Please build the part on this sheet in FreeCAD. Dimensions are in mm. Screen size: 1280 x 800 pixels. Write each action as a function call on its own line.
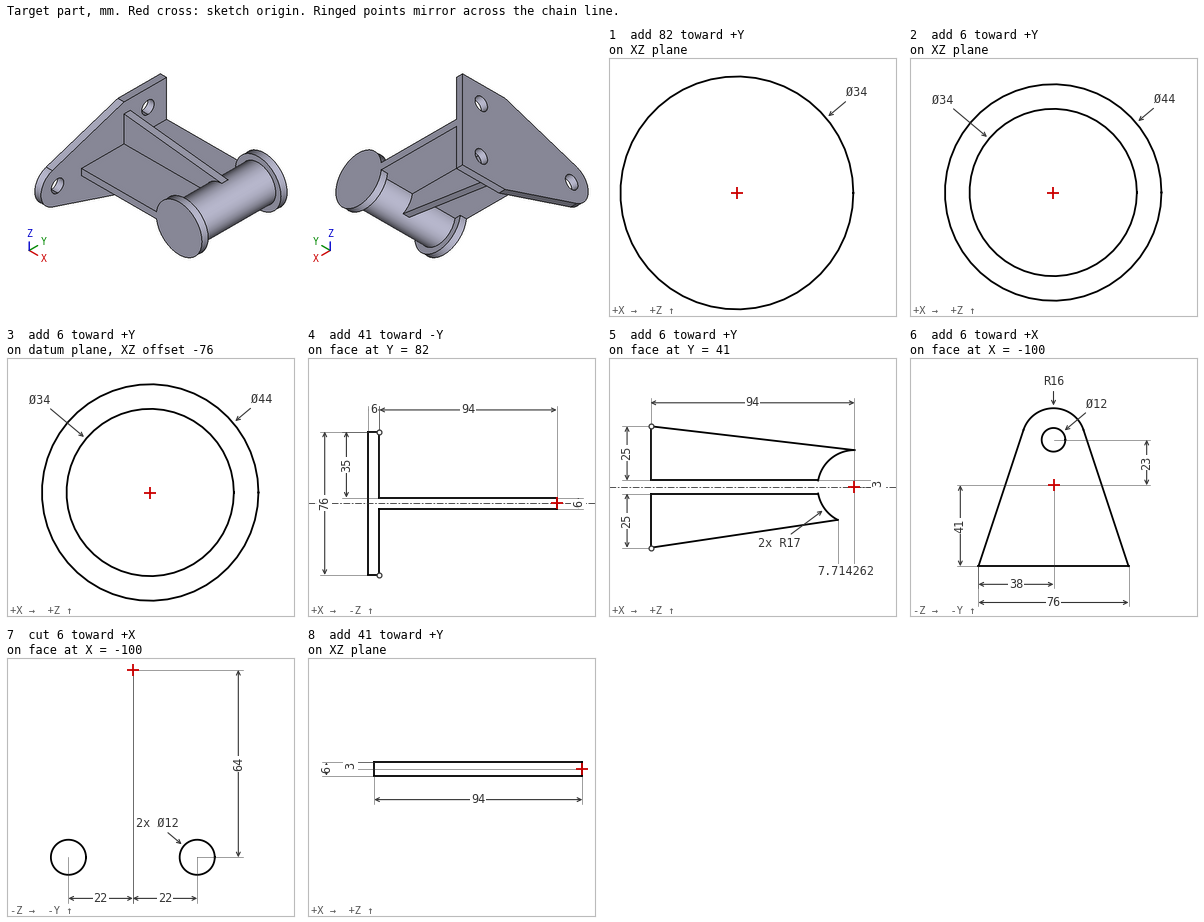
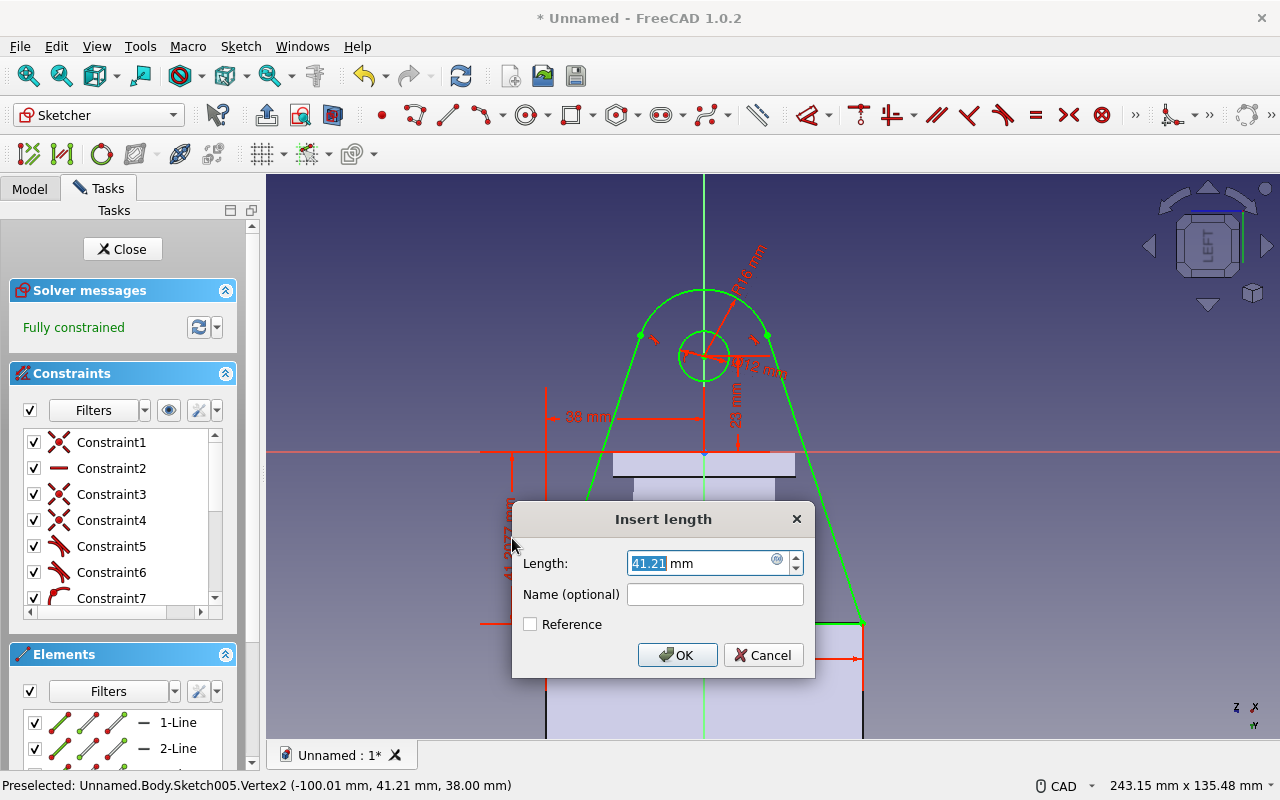
text(41)
key(Return)
key(Escape)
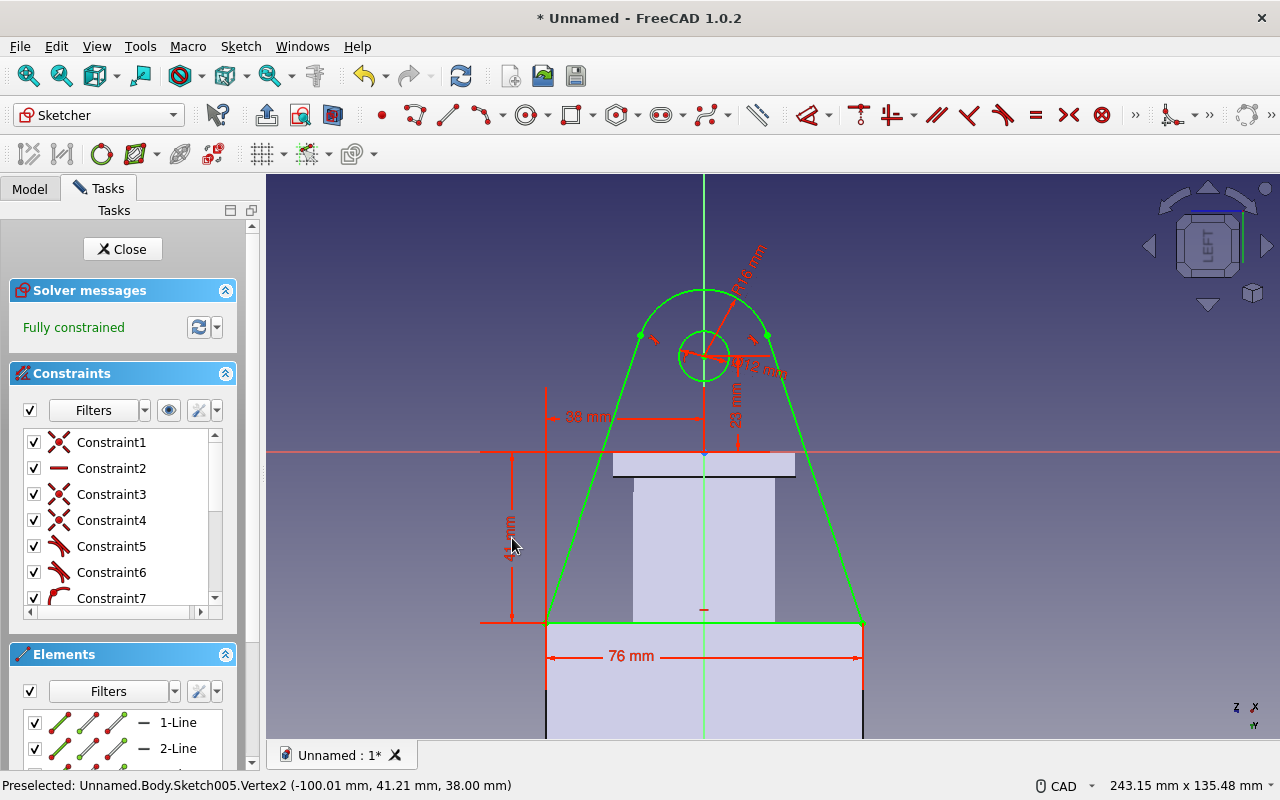
click(123, 249)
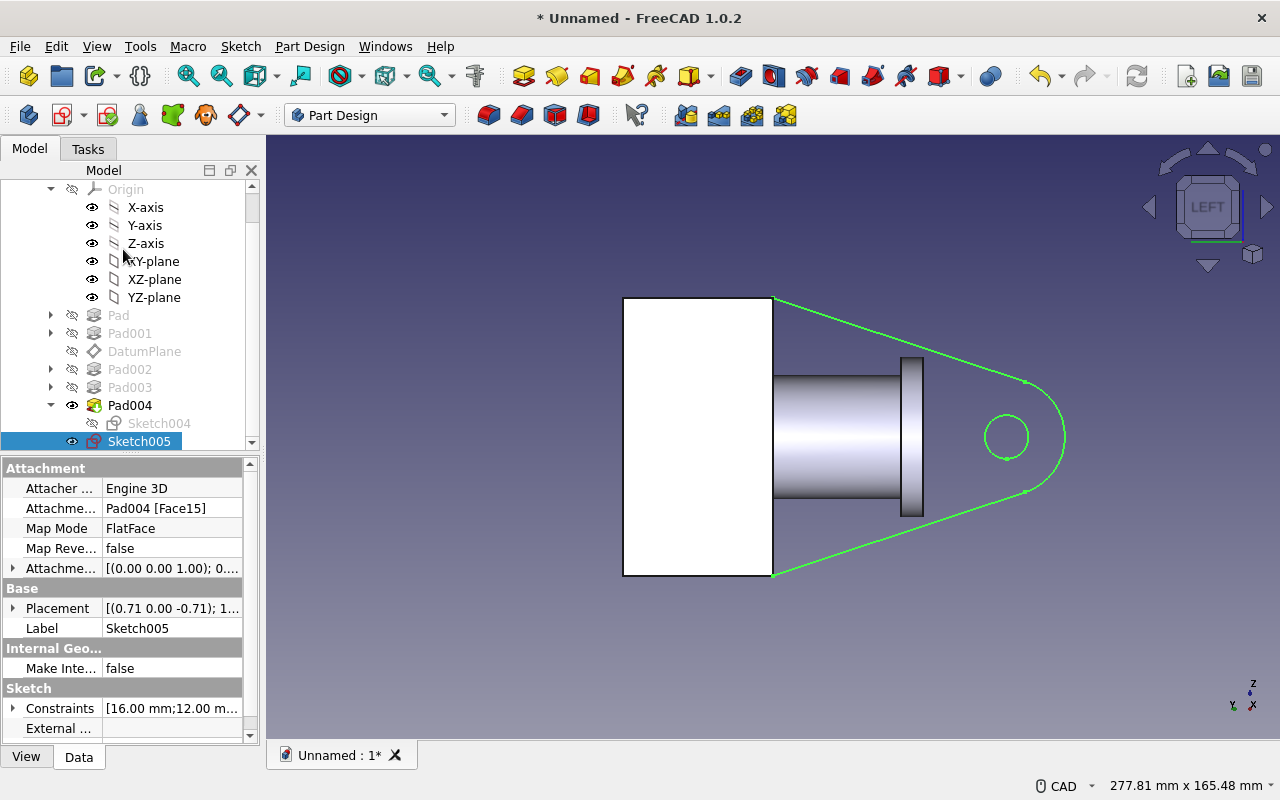
click(524, 76)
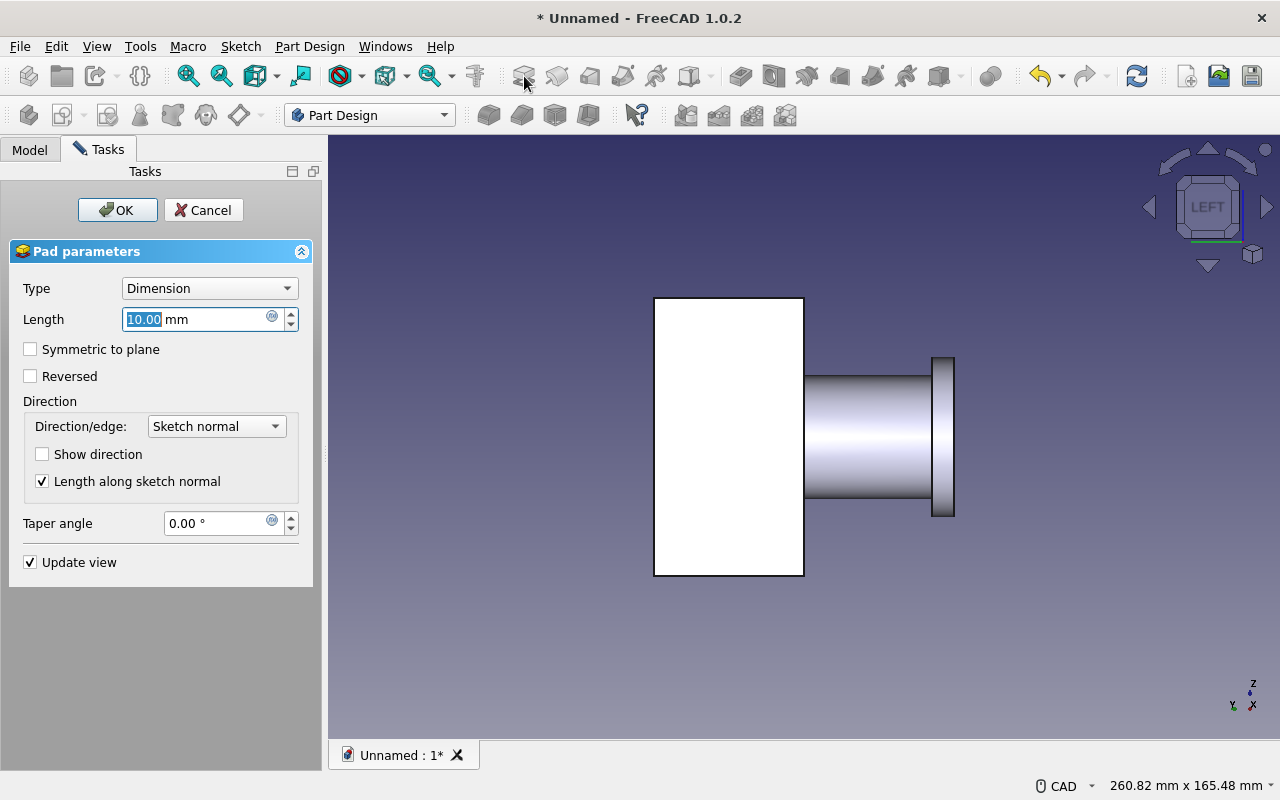
text(6)
key(Tab)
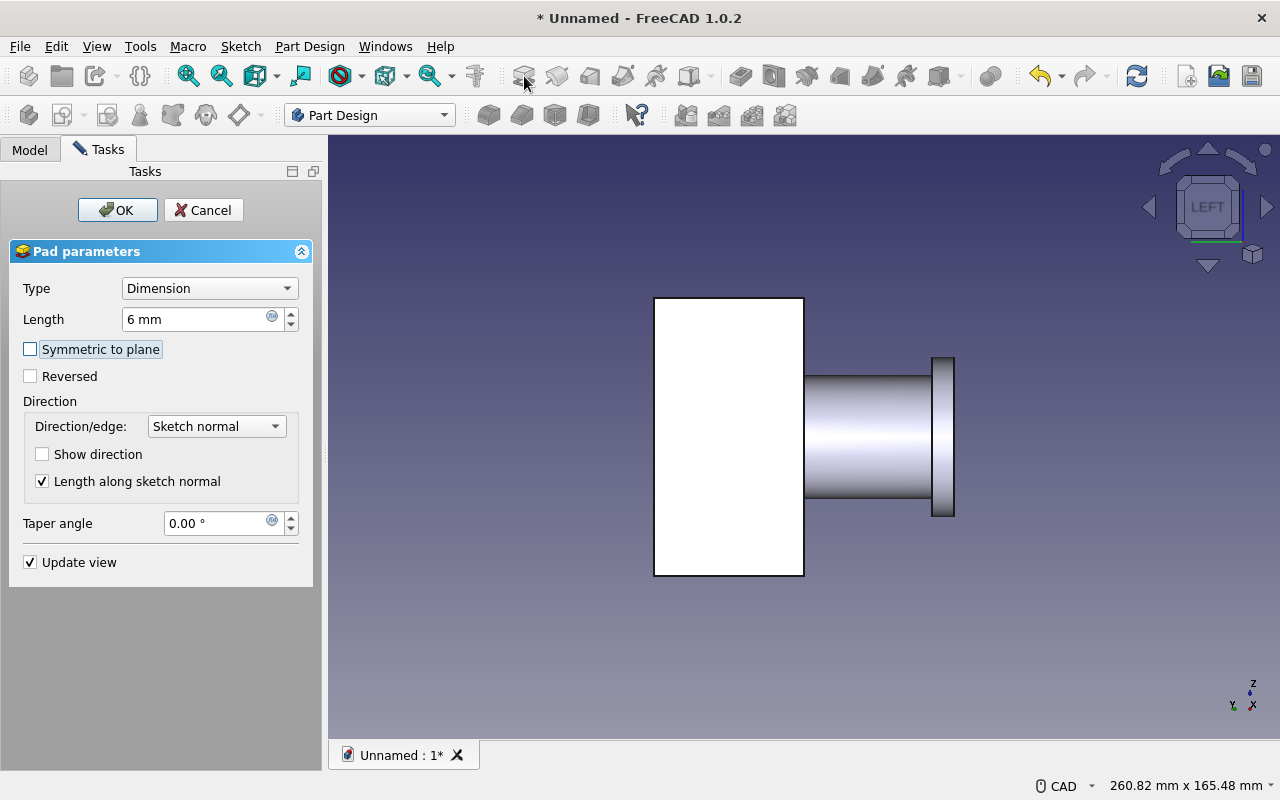
click(31, 376)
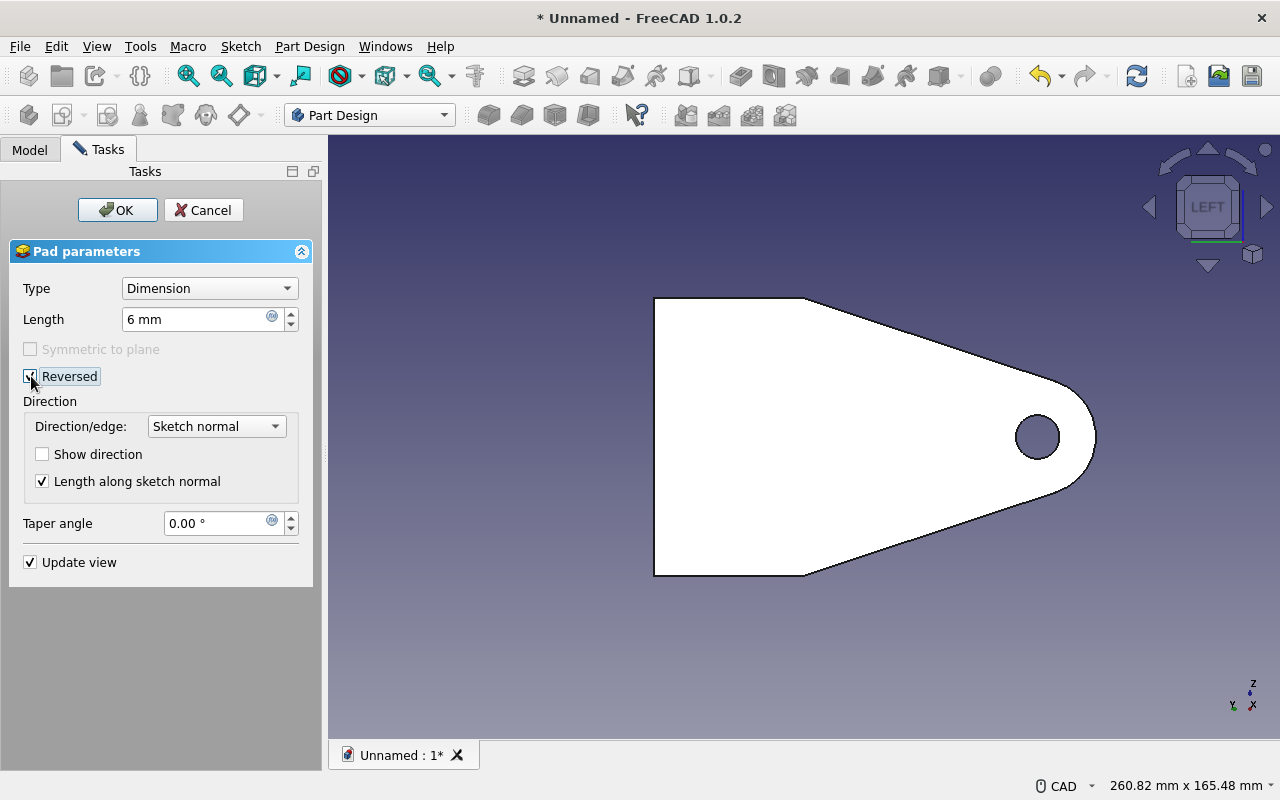
click(118, 210)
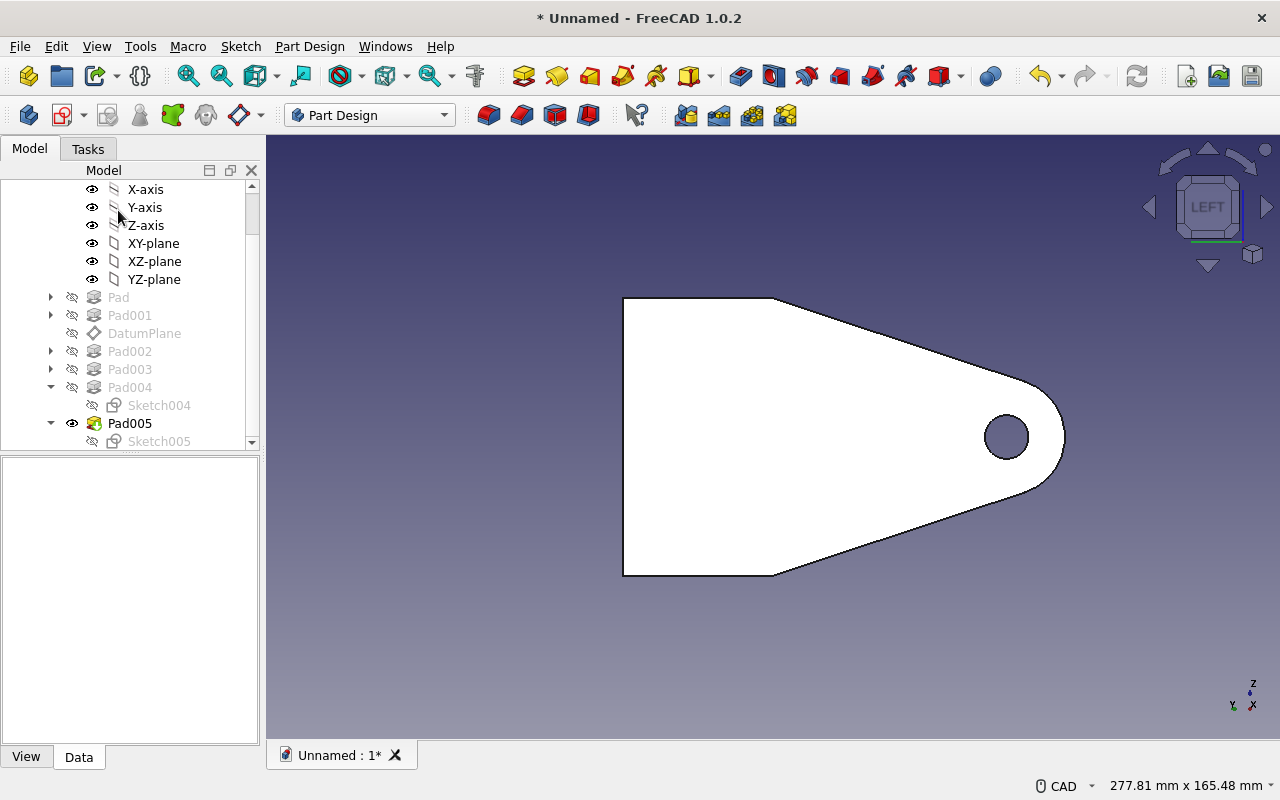
click(781, 436)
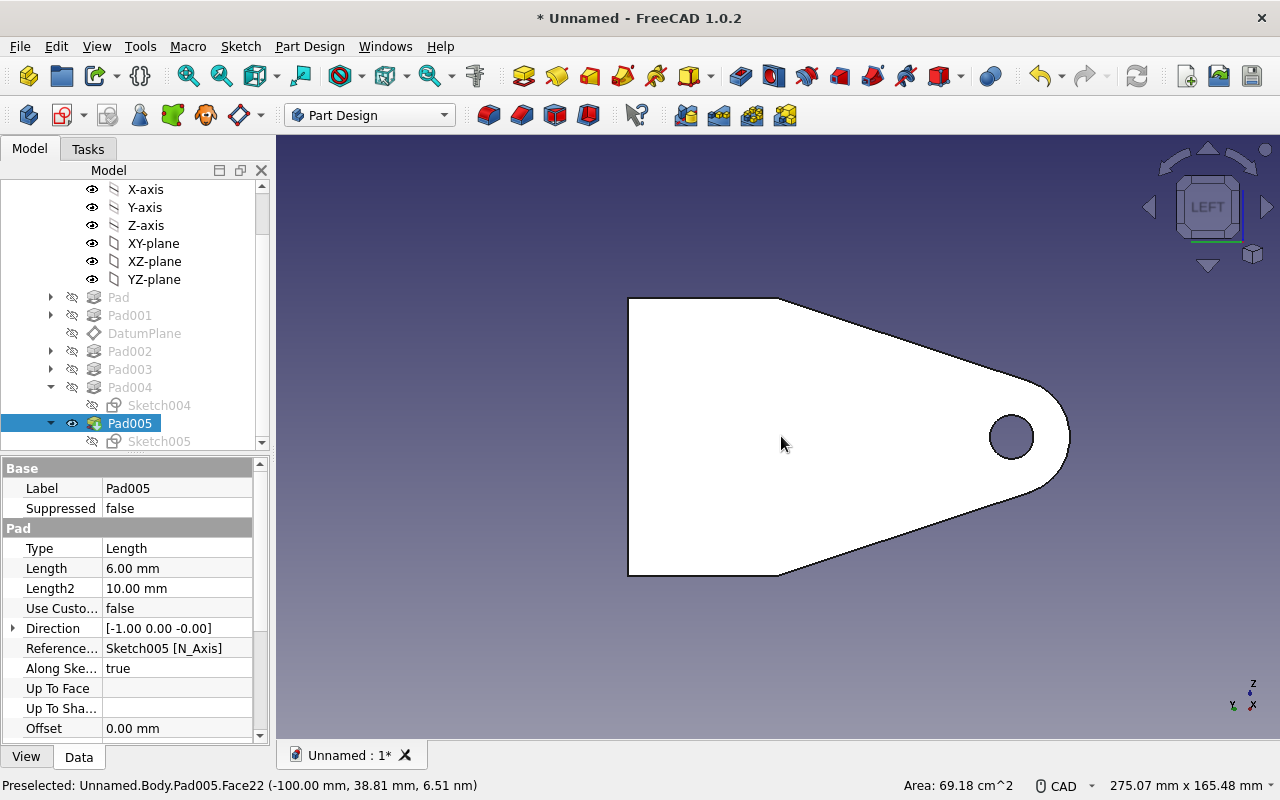
click(62, 116)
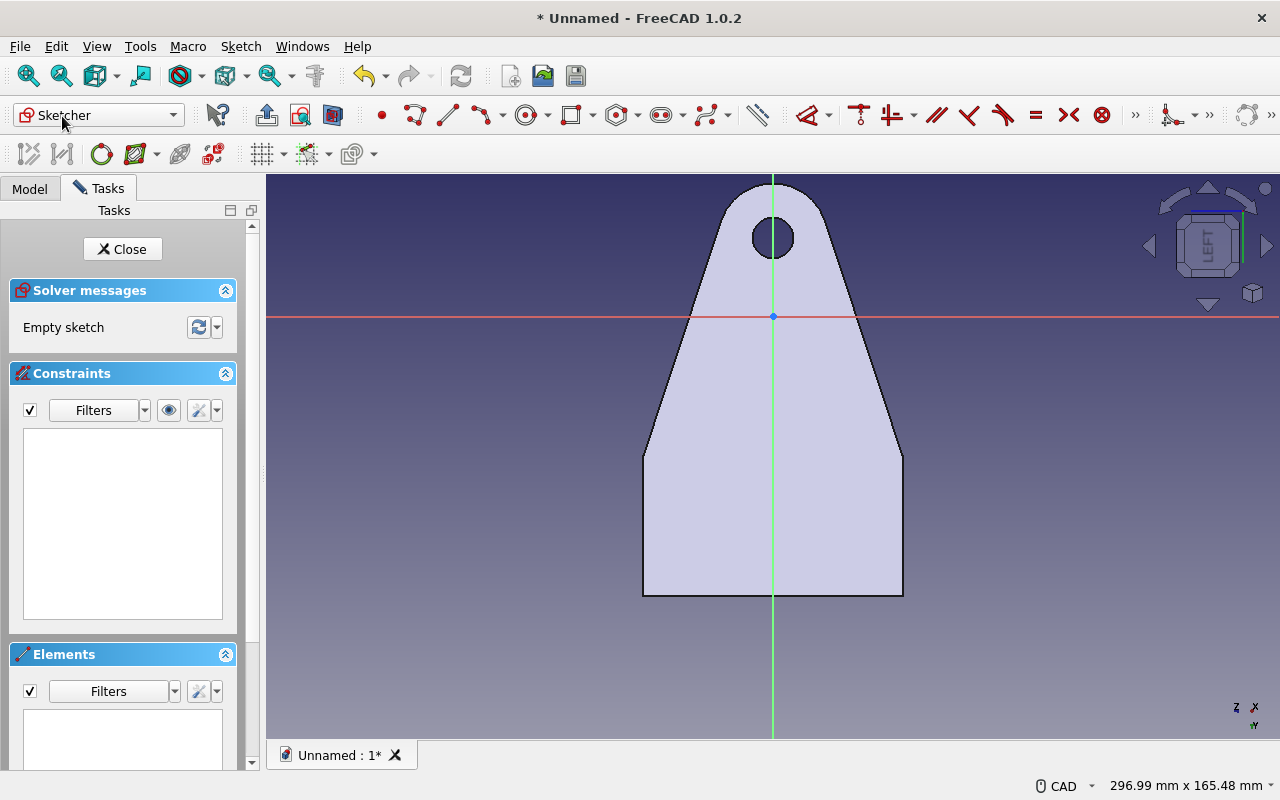
scroll(912, 394, up, 2)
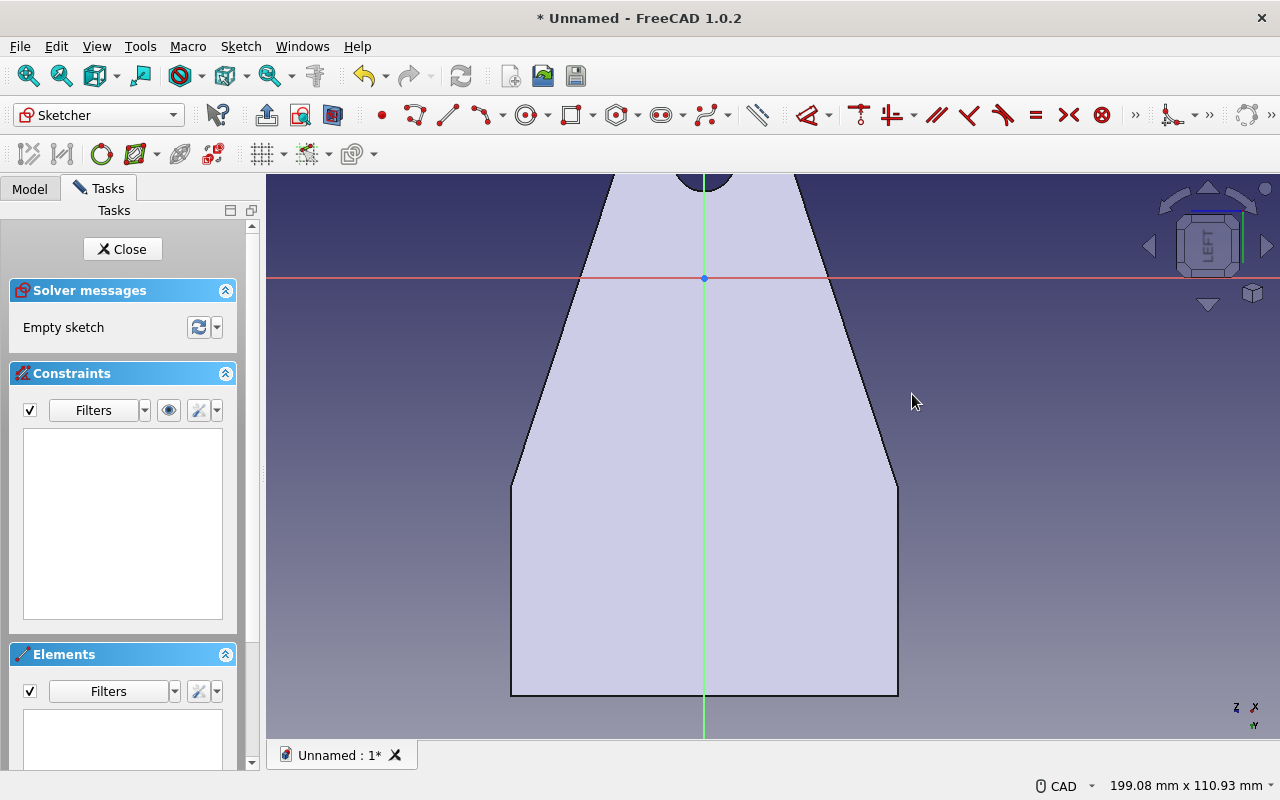
click(526, 116)